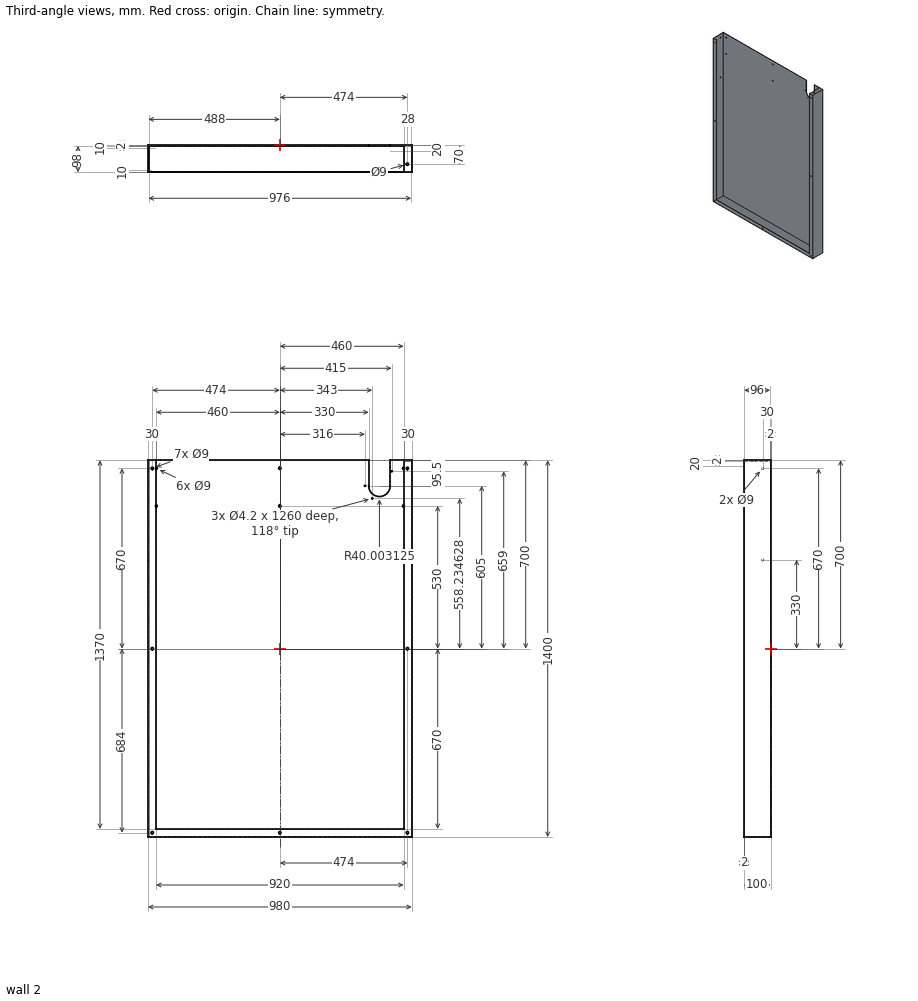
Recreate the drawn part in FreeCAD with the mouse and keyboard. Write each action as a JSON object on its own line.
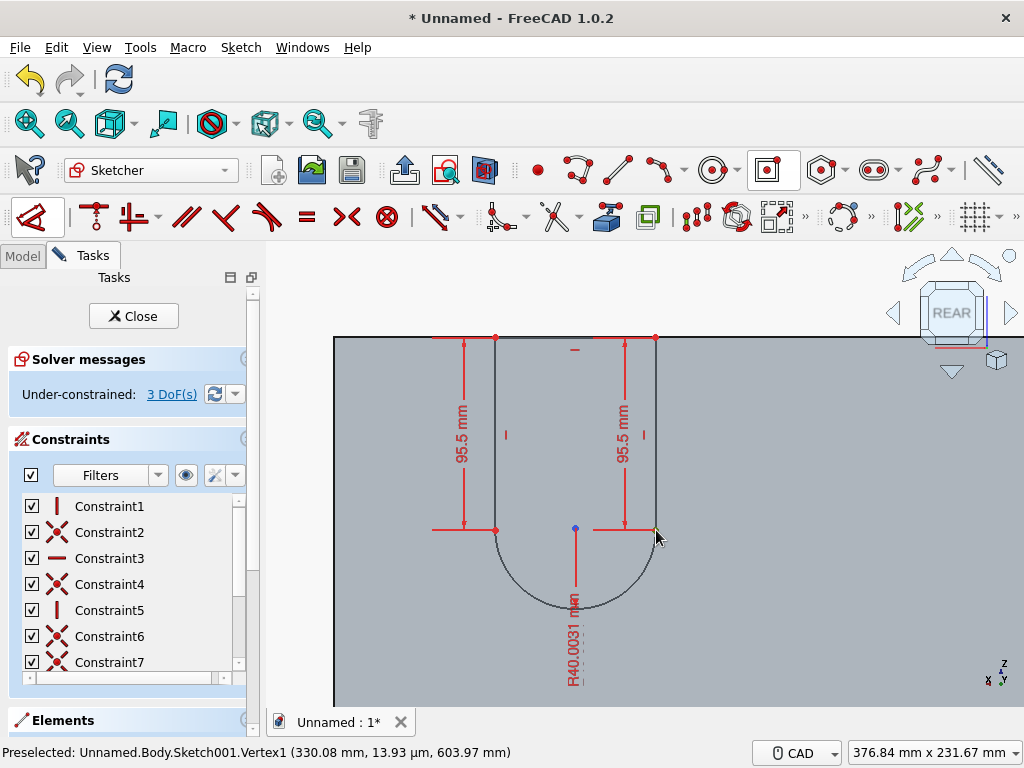
{"action": "left_click", "coordinate": [58, 218]}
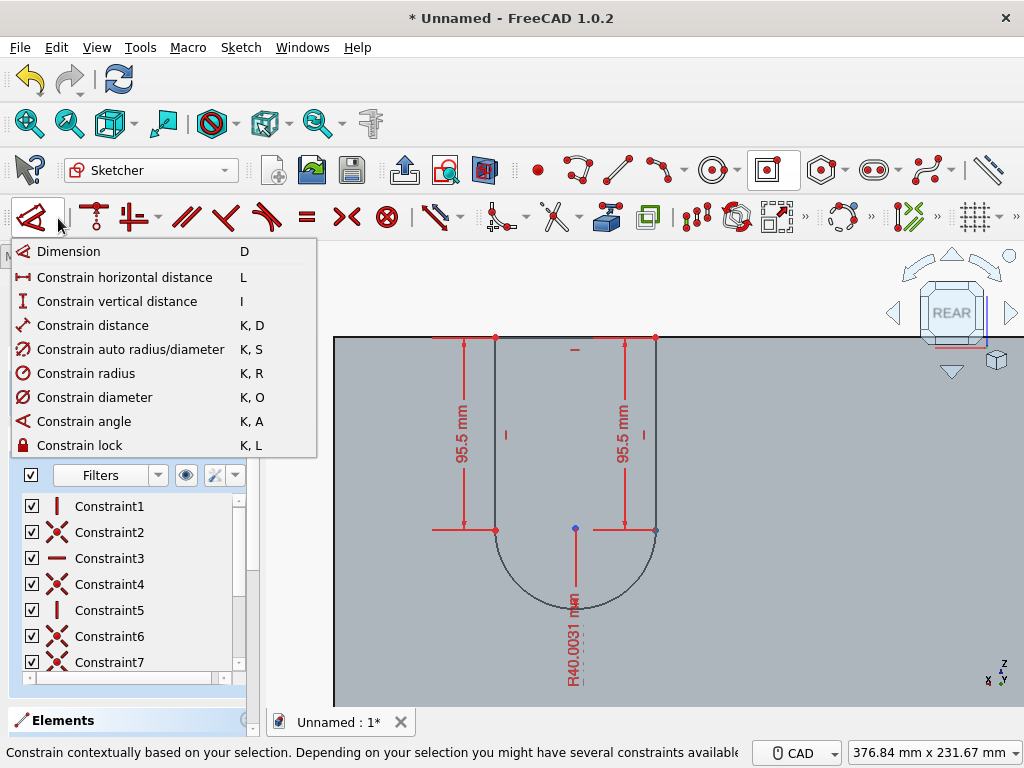
{"action": "left_click", "coordinate": [164, 277]}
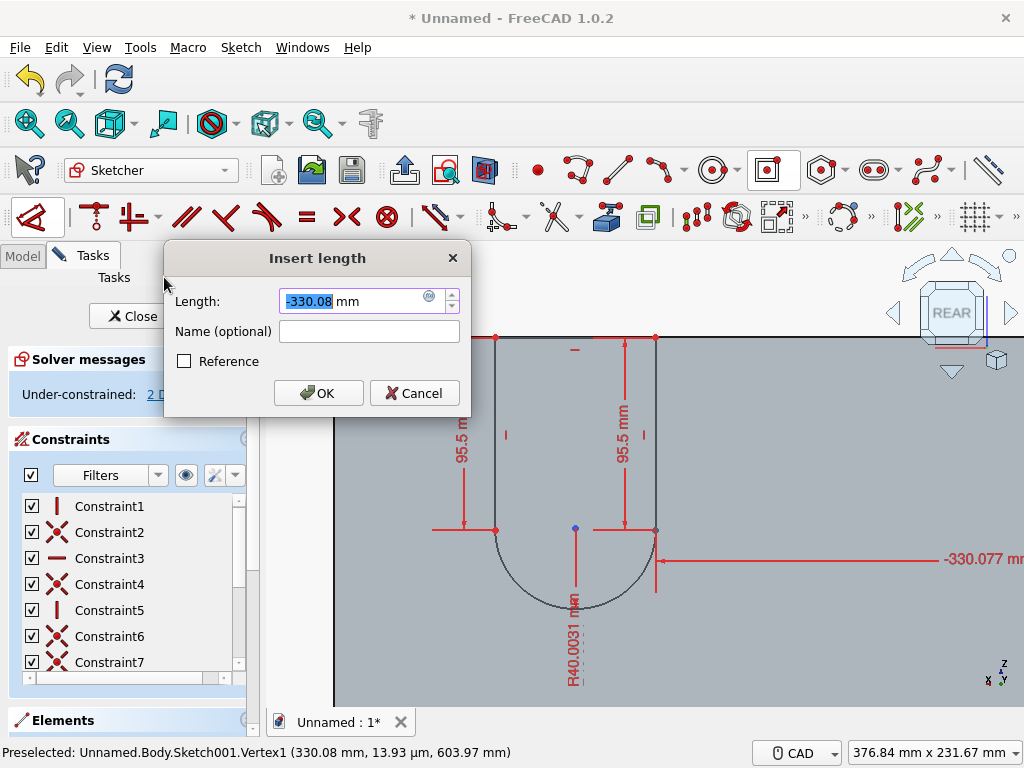
{"action": "type", "text": "-330"}
{"action": "key", "text": "Return"}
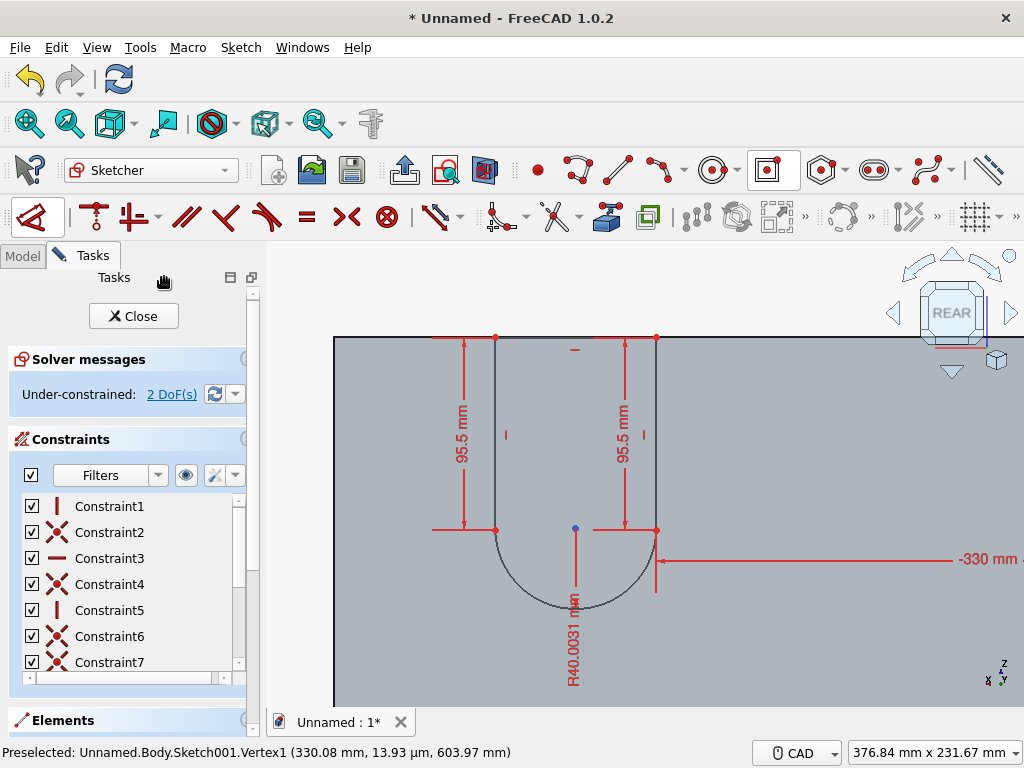
{"action": "left_click", "coordinate": [656, 338]}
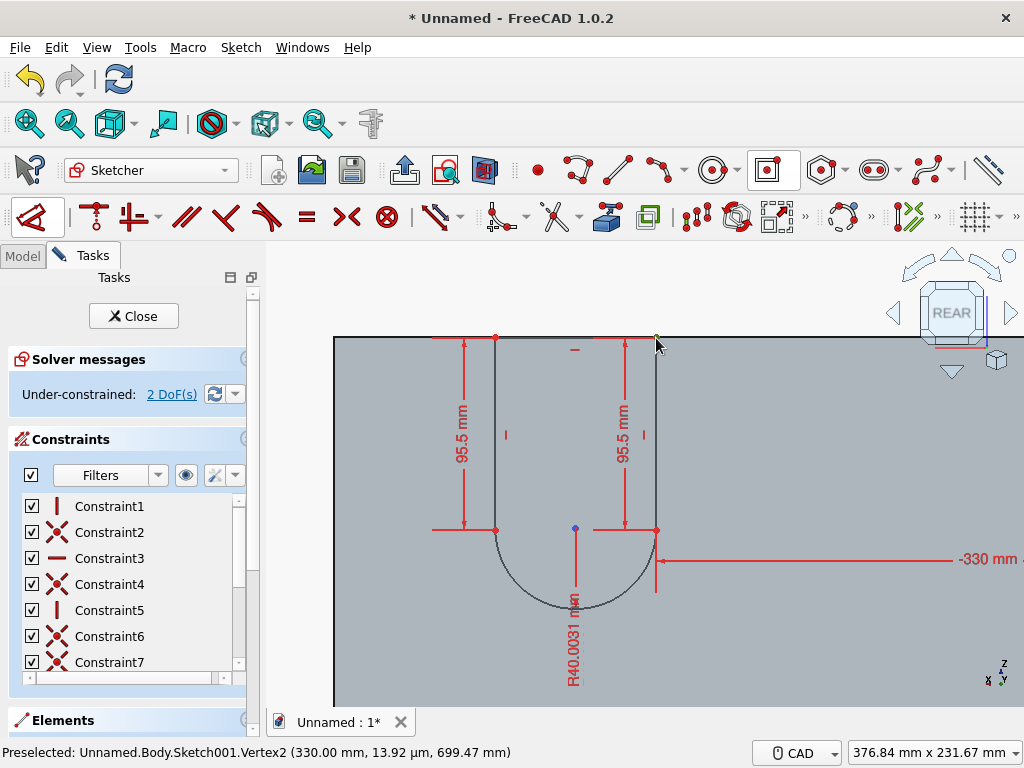
{"action": "key", "text": "i"}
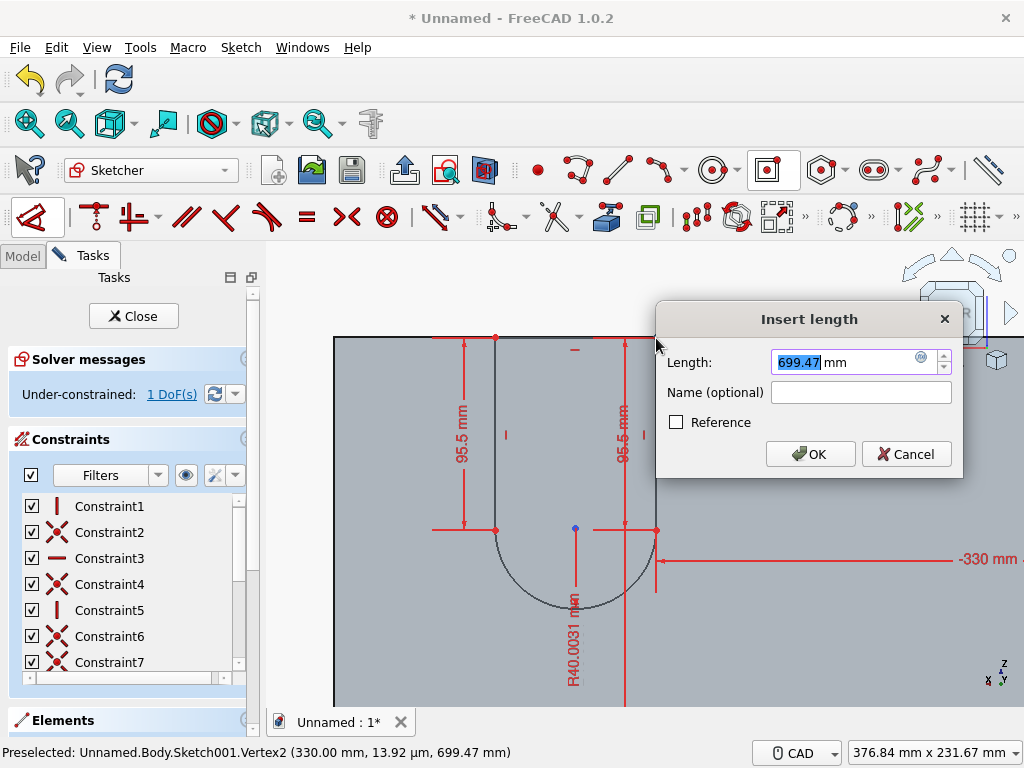
{"action": "type", "text": "700"}
{"action": "key", "text": "Return"}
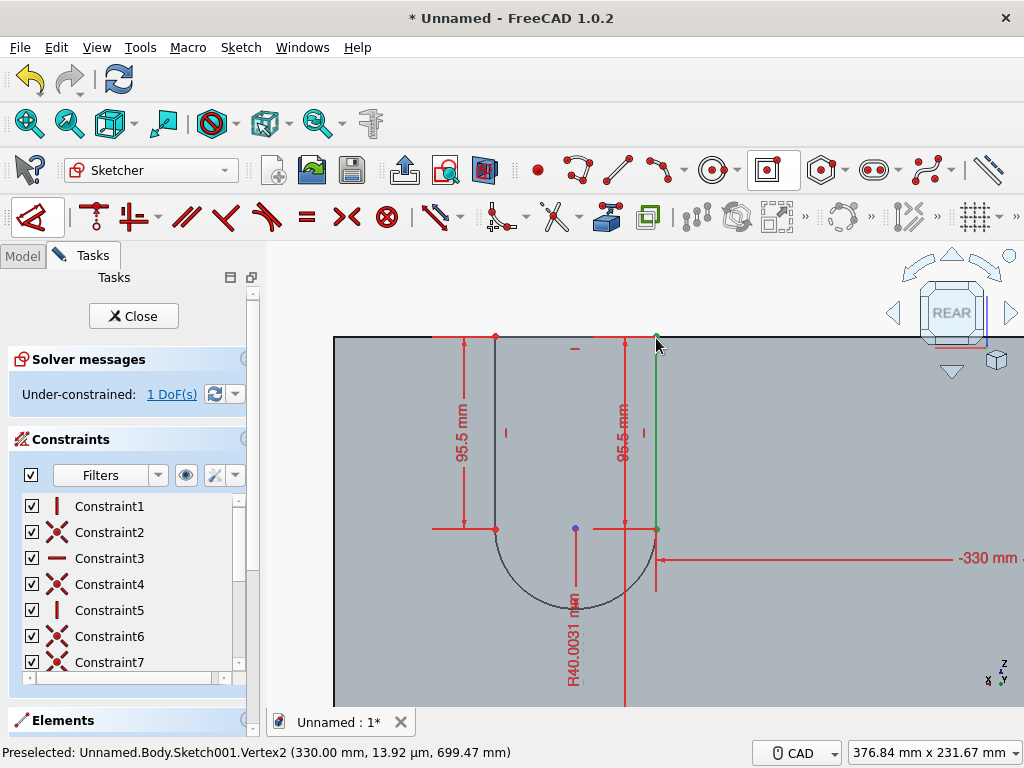
{"action": "left_click", "coordinate": [576, 528]}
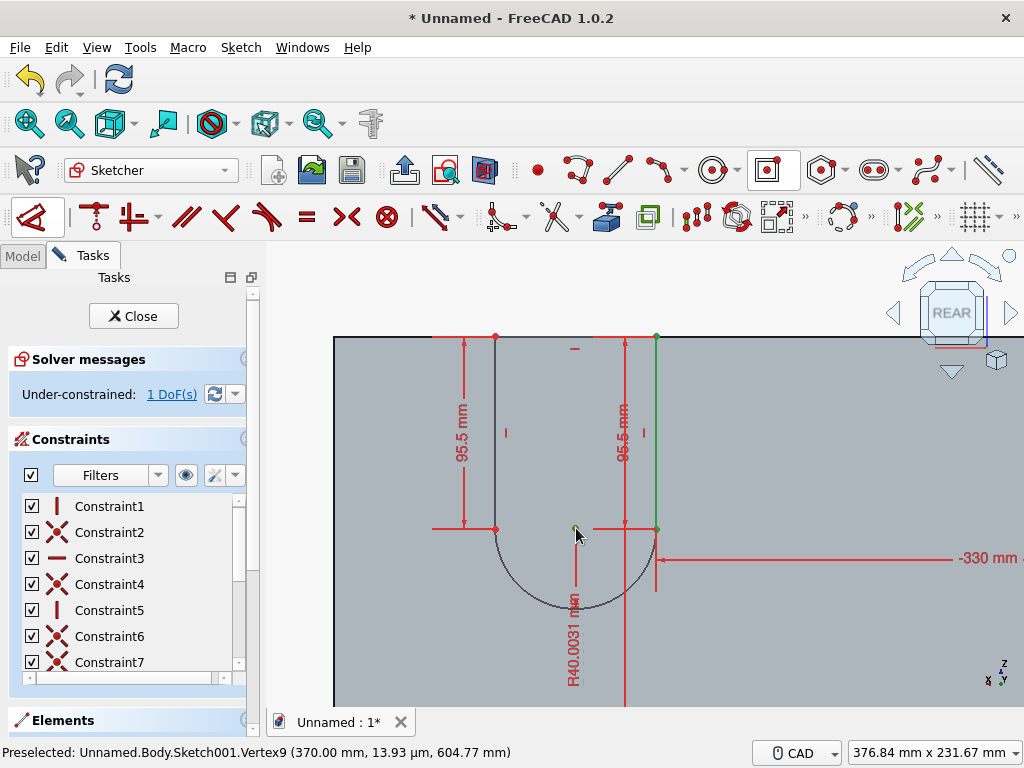
{"action": "key", "text": "i"}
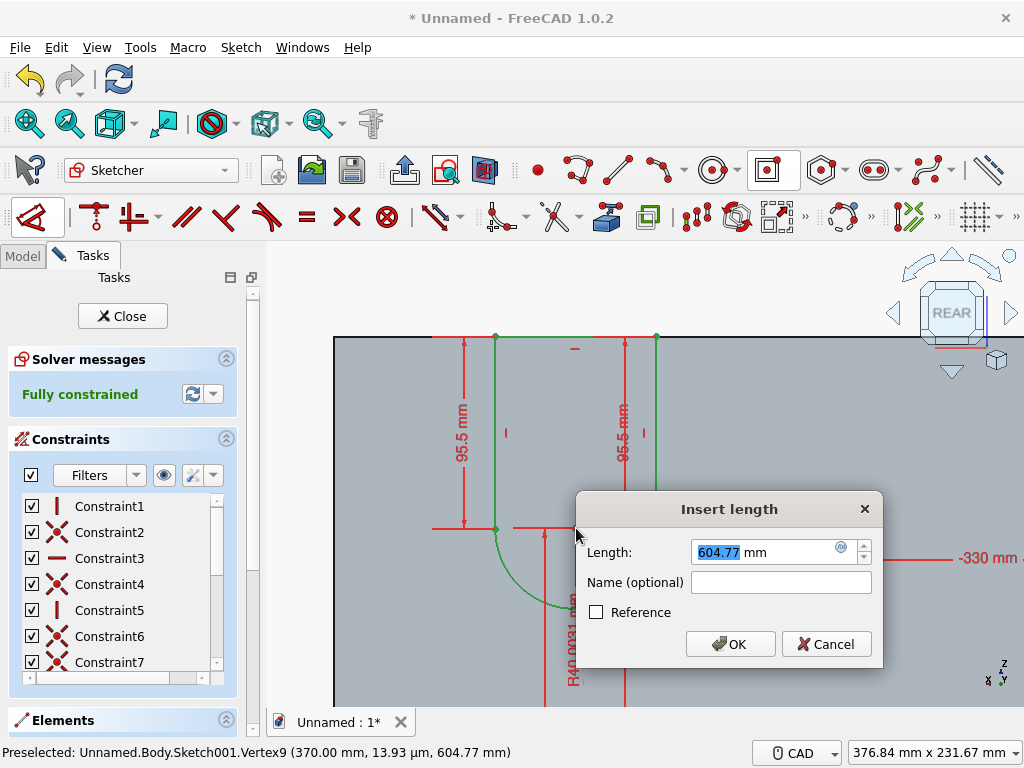
{"action": "type", "text": "605"}
{"action": "key", "text": "Return"}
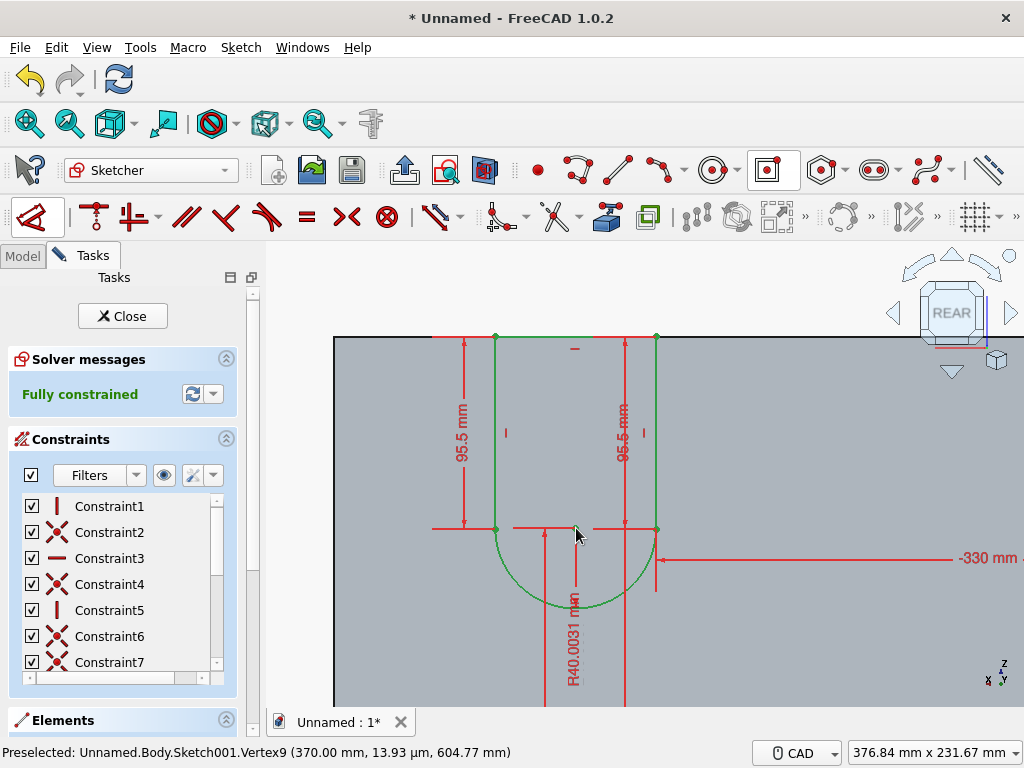
{"action": "left_click", "coordinate": [123, 316]}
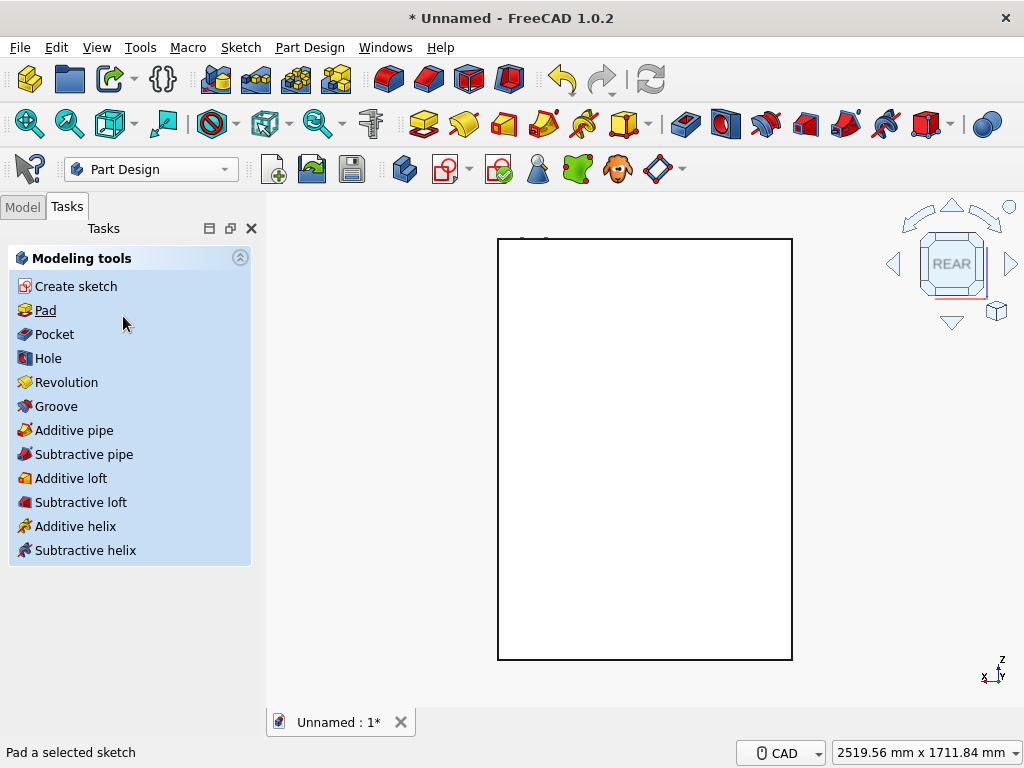
{"action": "left_click", "coordinate": [686, 124]}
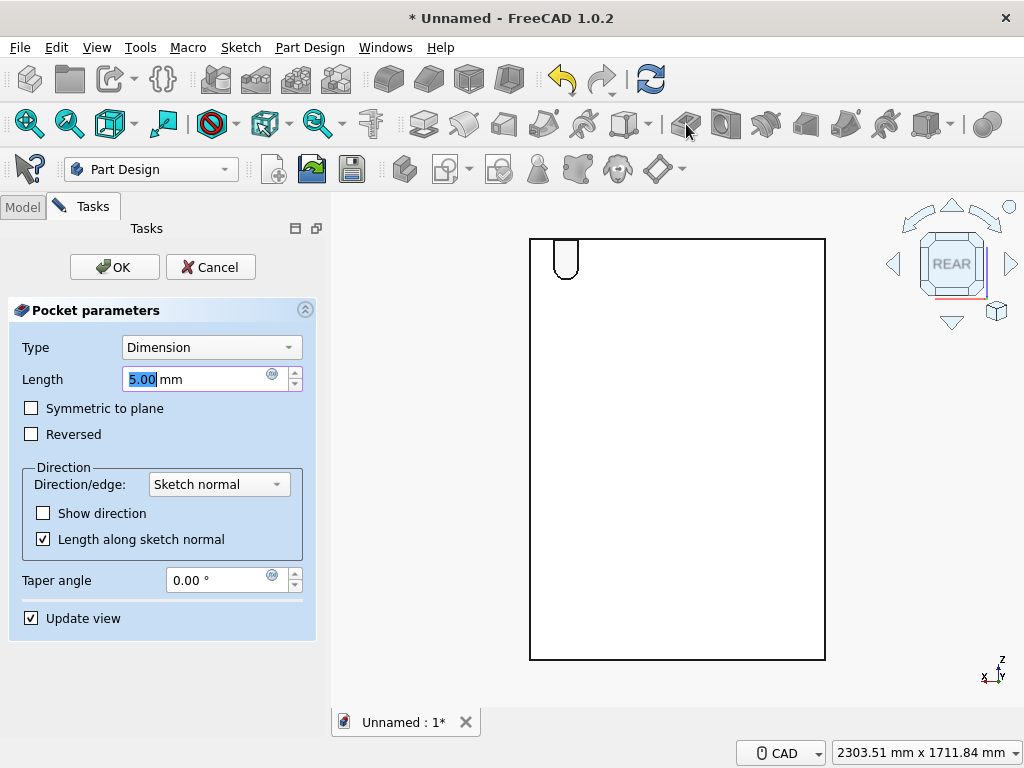
{"action": "type", "text": "20"}
{"action": "key", "text": "Tab"}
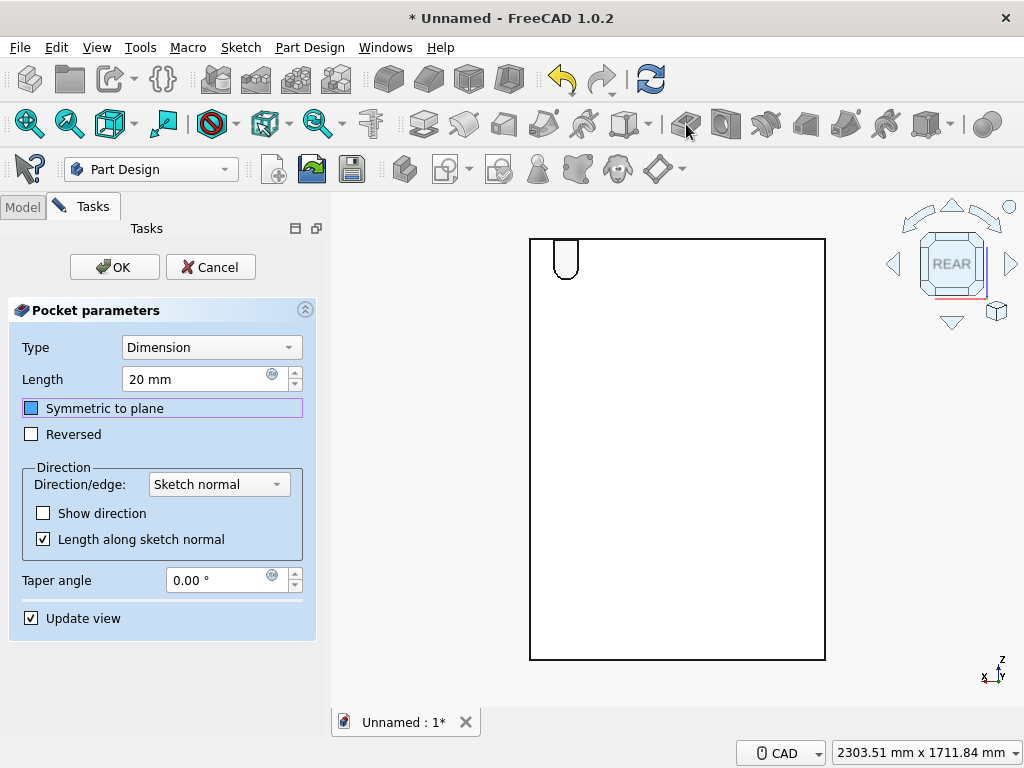
{"action": "left_click", "coordinate": [115, 267]}